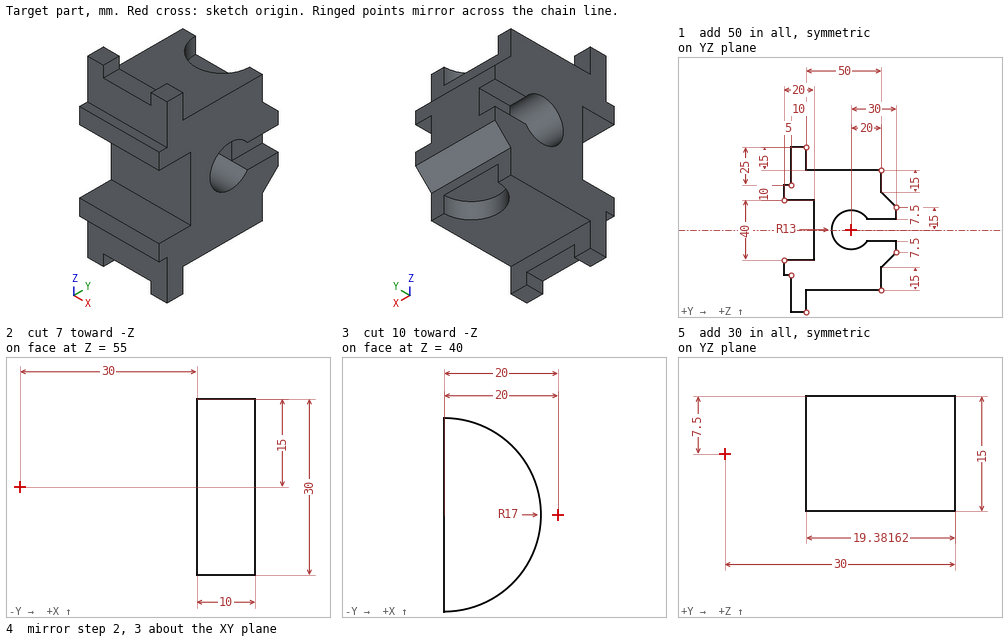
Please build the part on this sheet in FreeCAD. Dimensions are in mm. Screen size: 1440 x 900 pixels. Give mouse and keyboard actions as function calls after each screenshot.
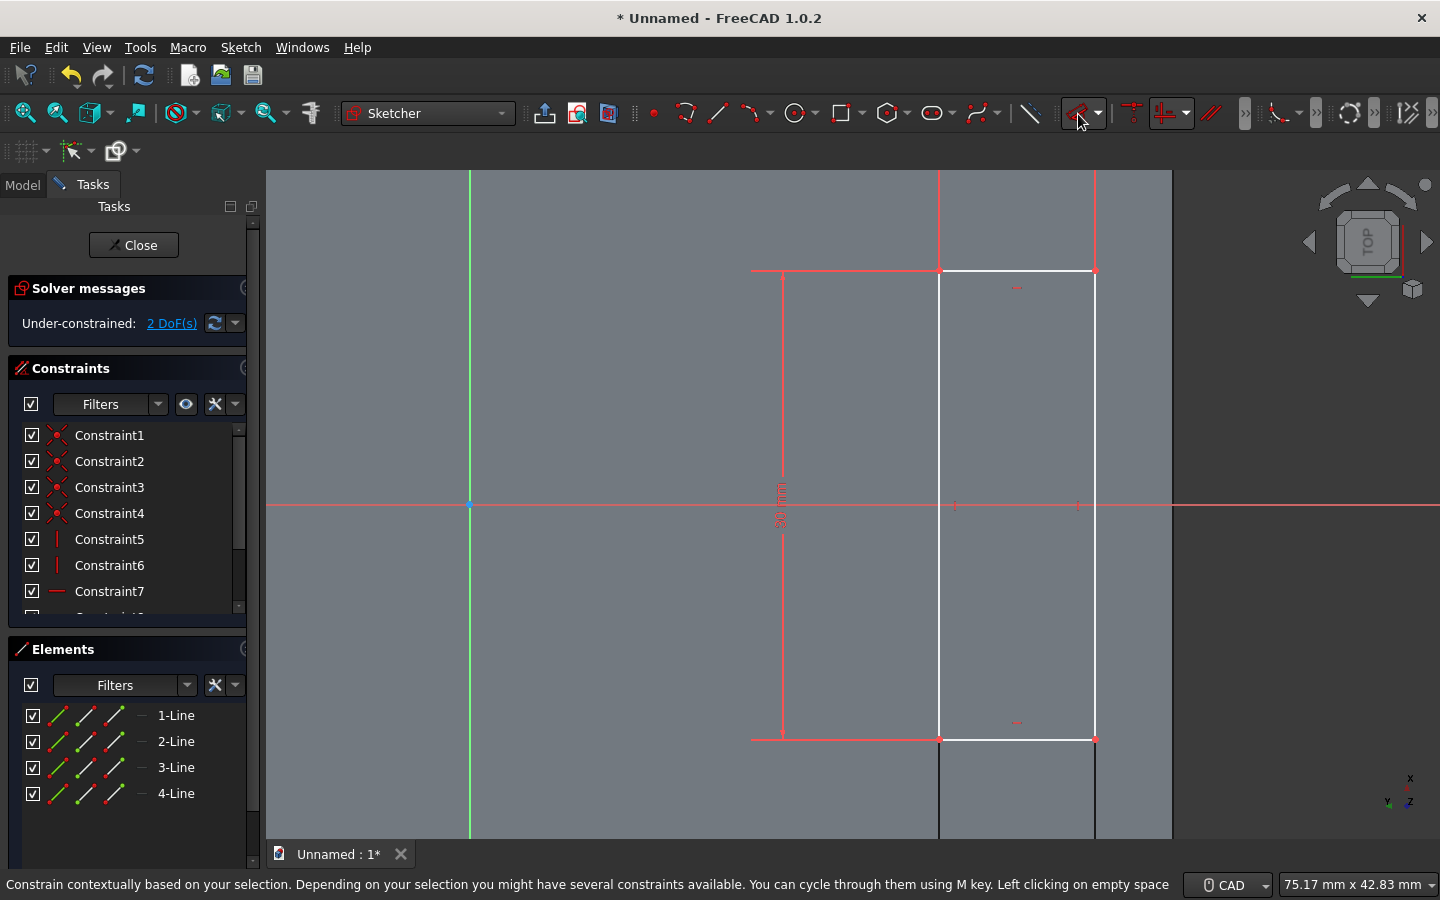
click(939, 271)
click(704, 237)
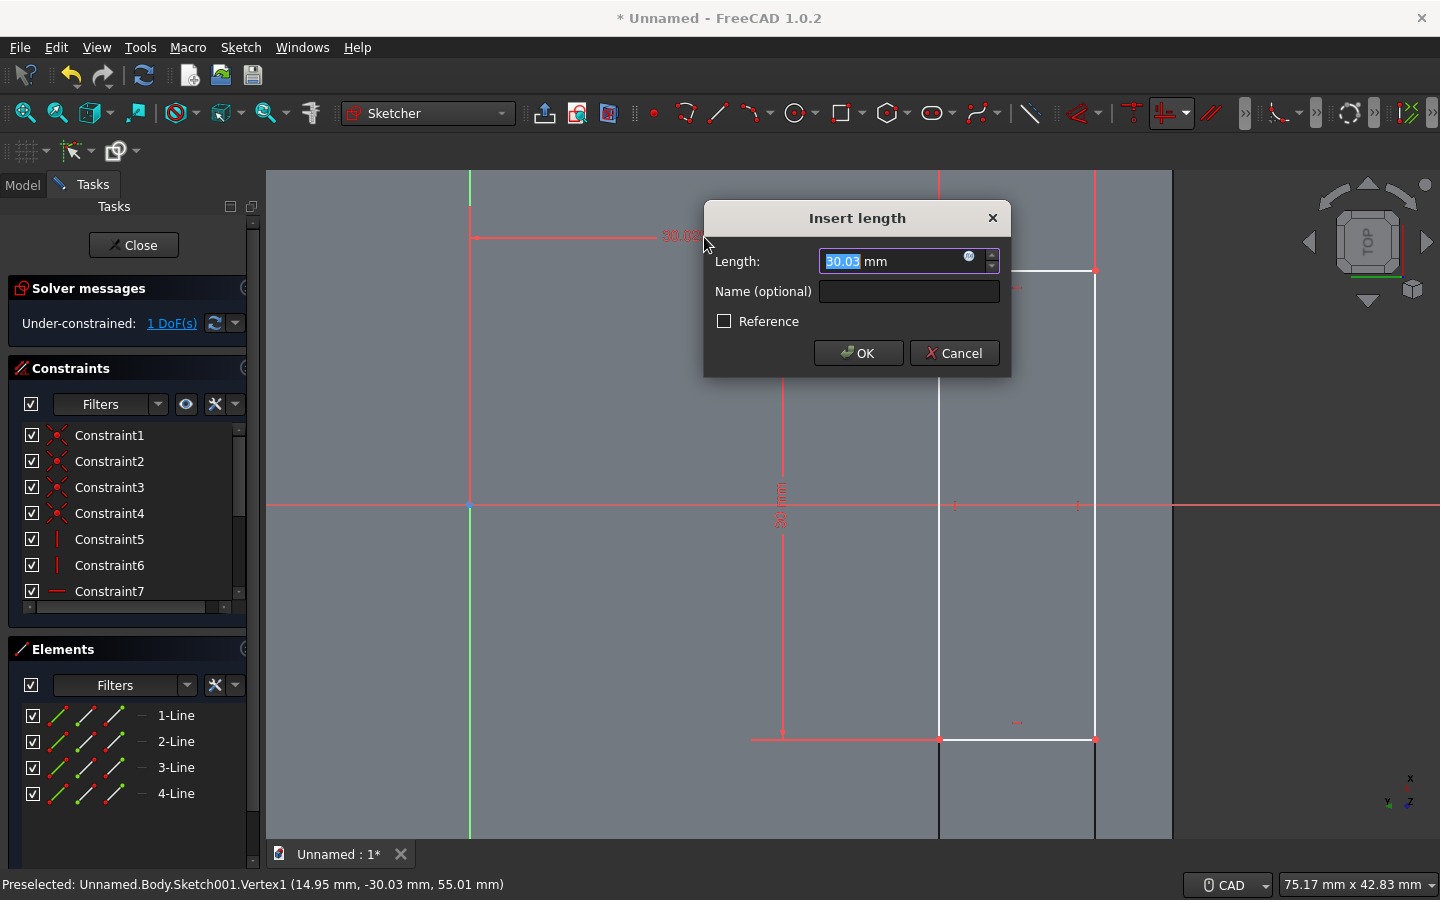
text(30)
key(Return)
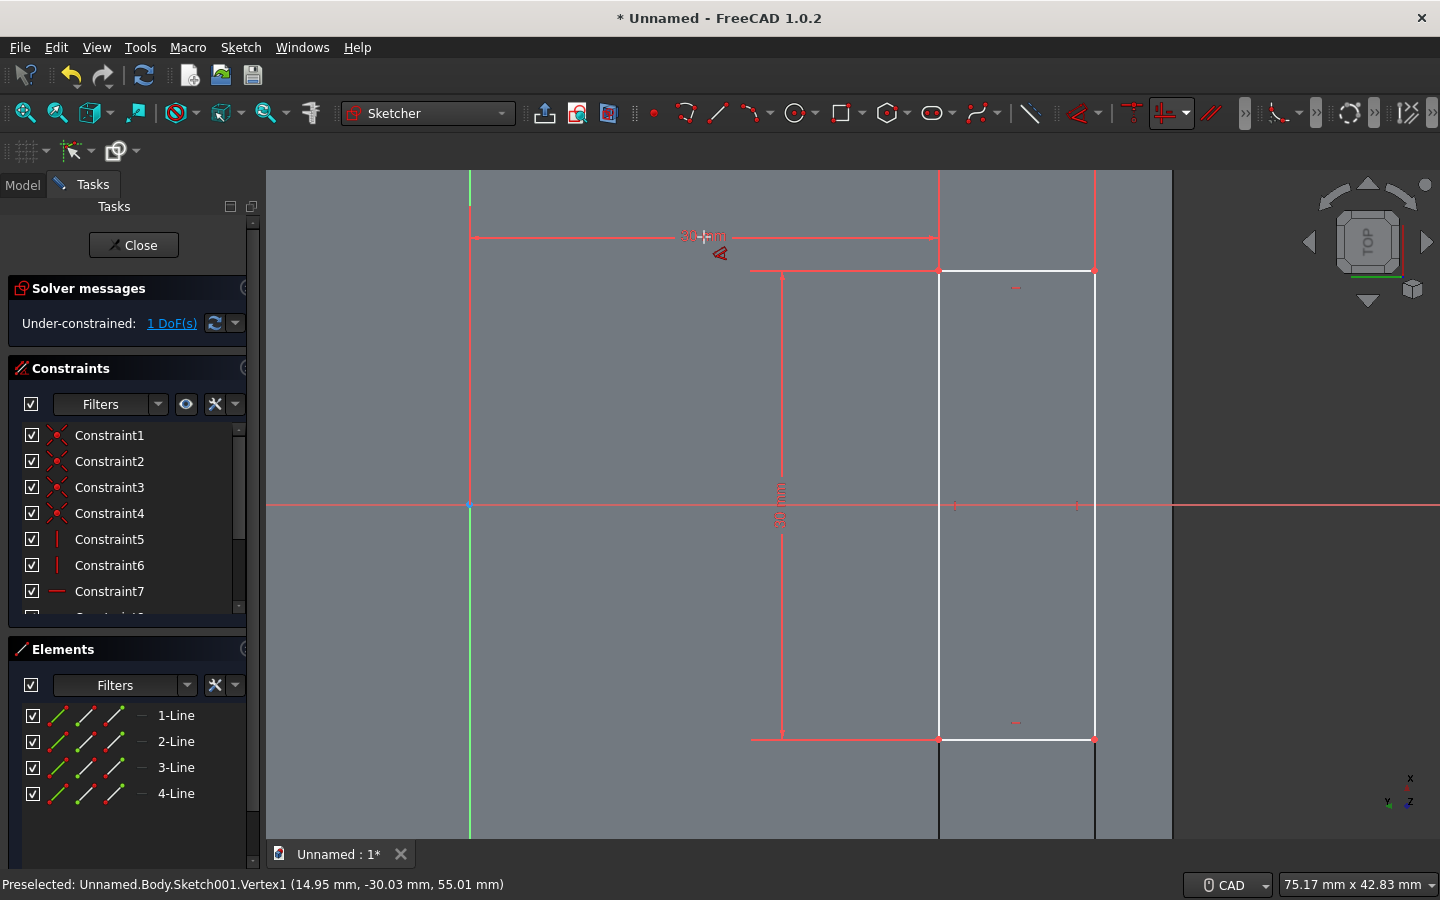
click(939, 271)
click(436, 388)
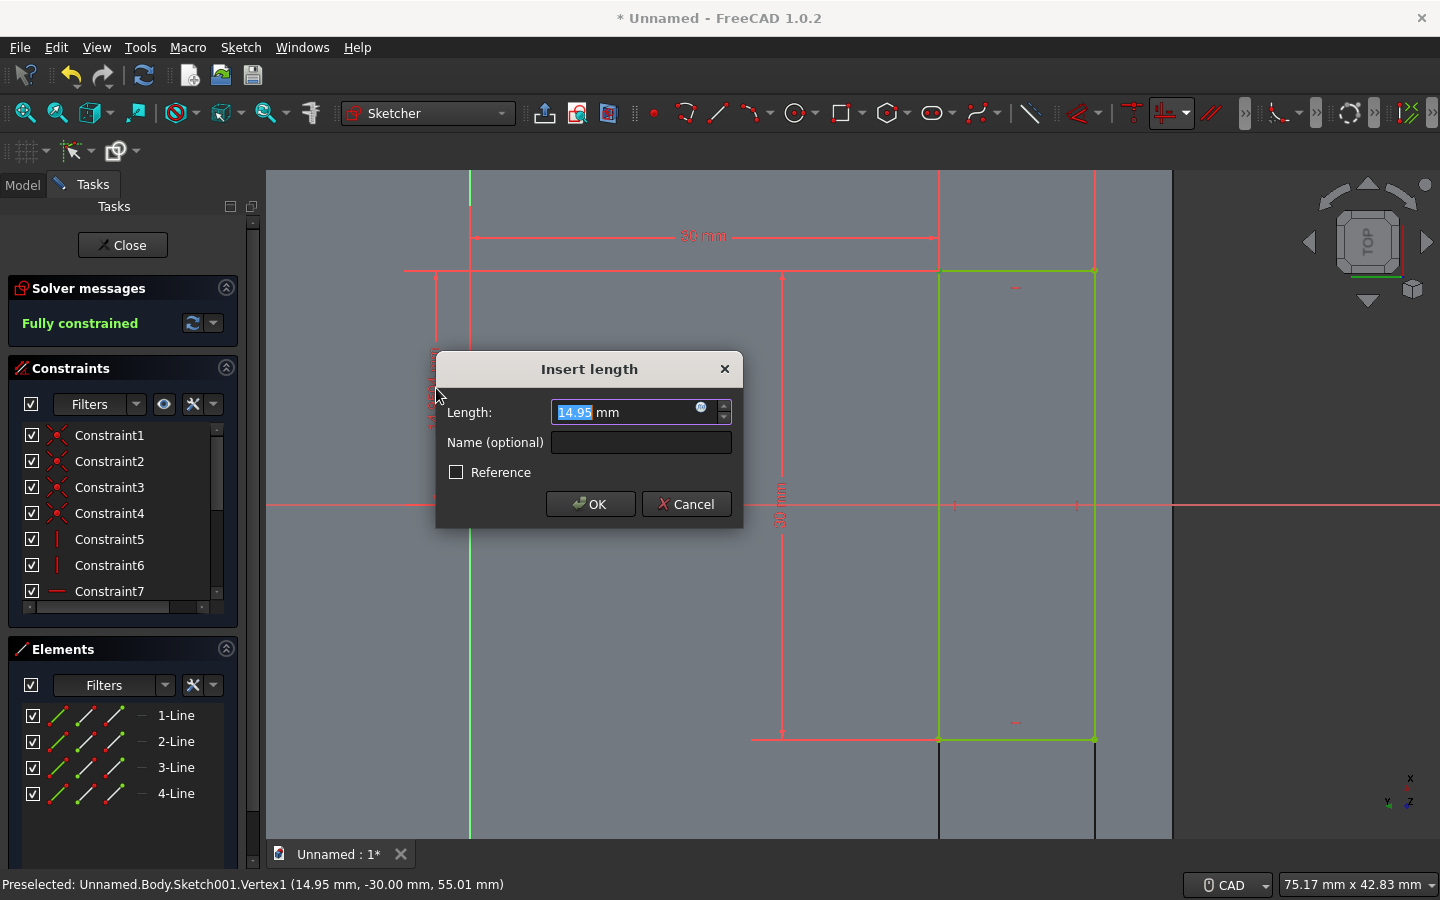
text(15)
key(Return)
key(Escape)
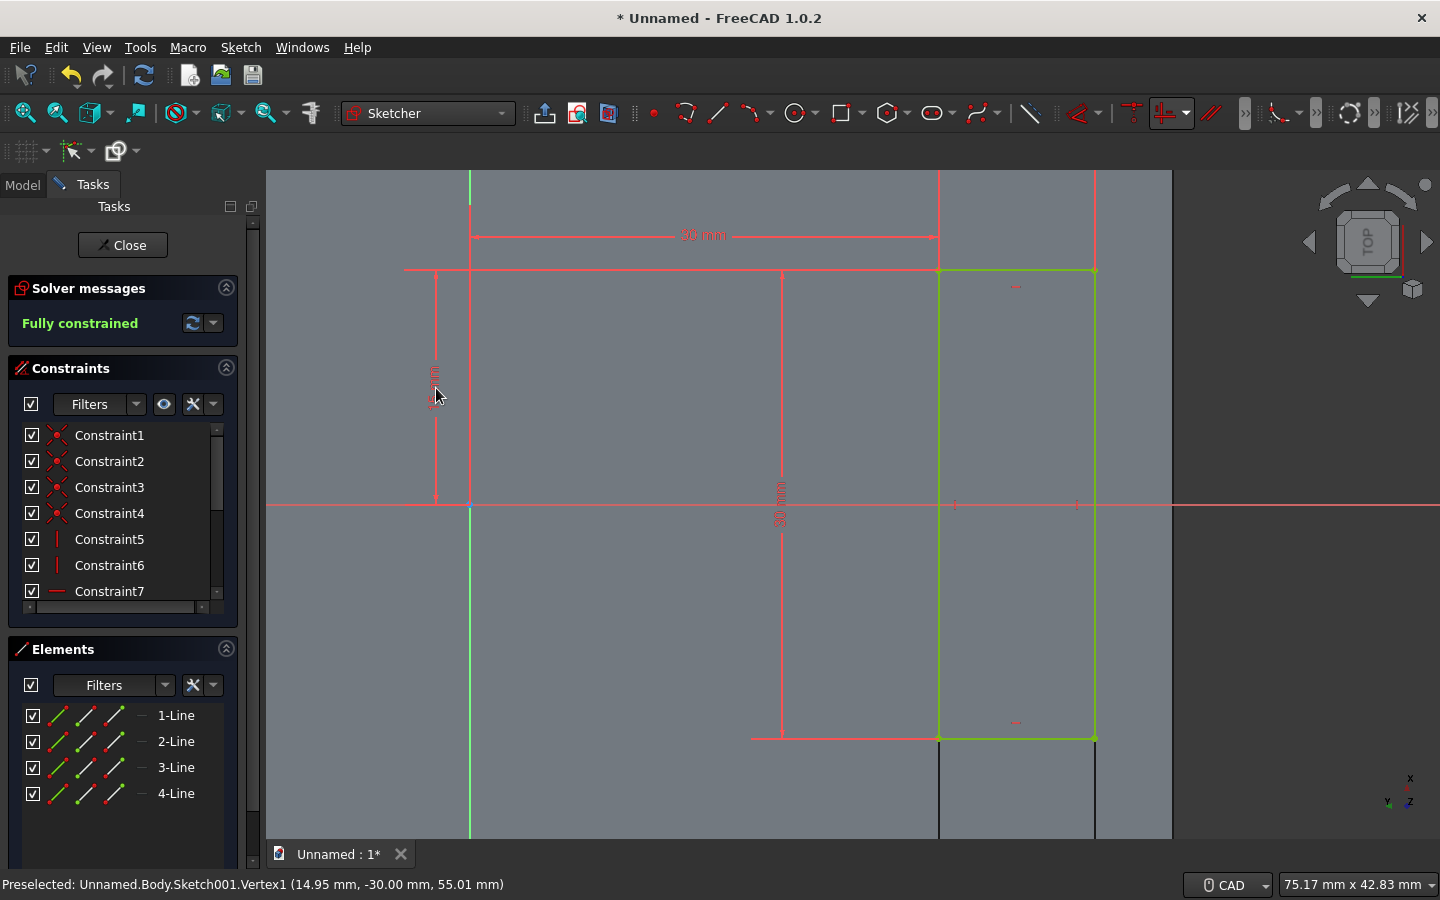
click(123, 245)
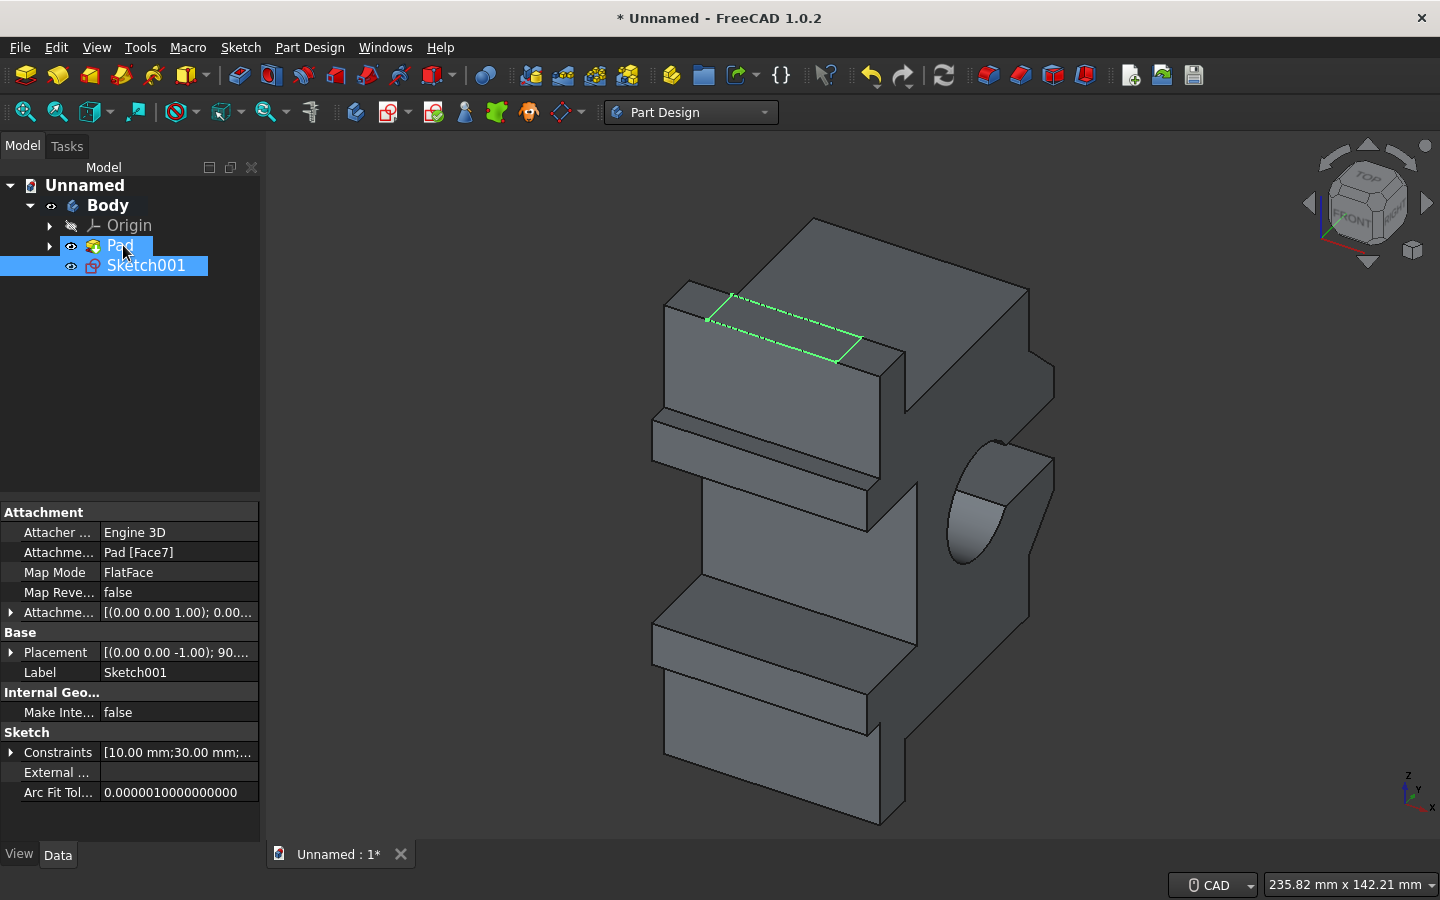
click(240, 76)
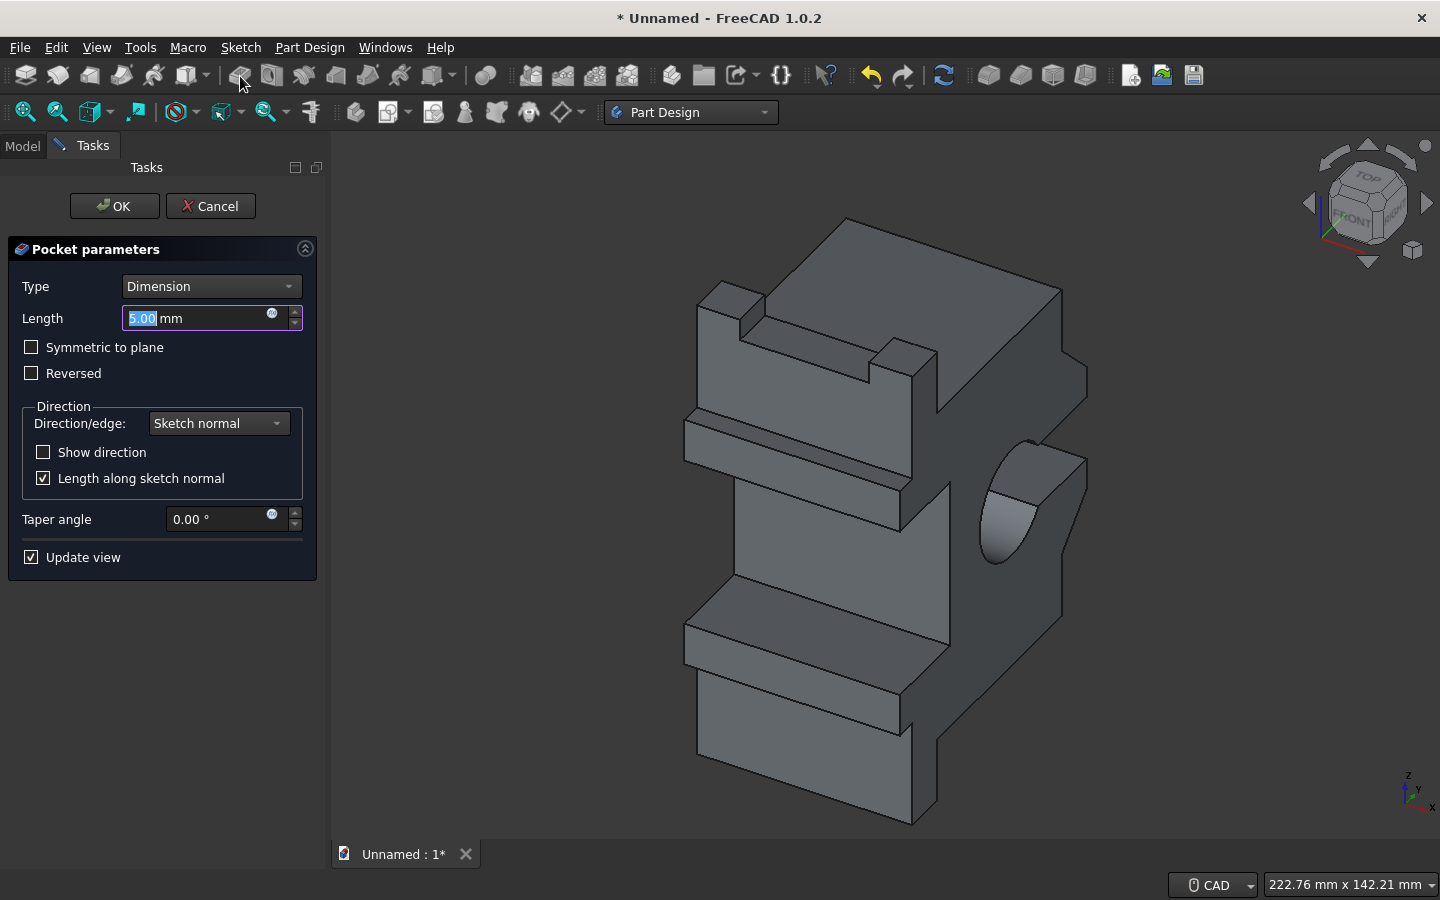
text(7)
key(Tab)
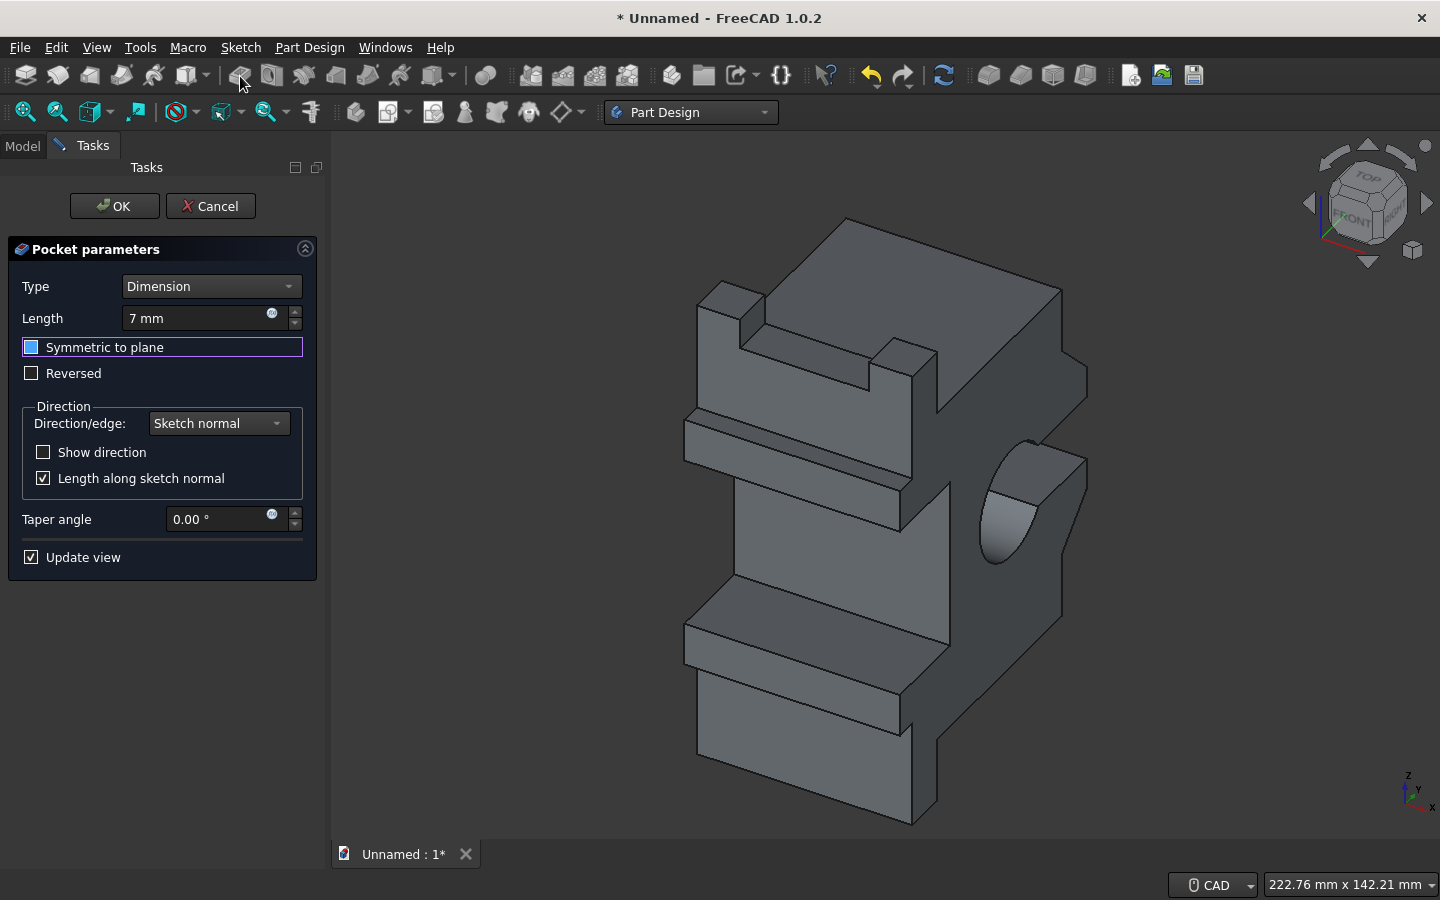
click(115, 206)